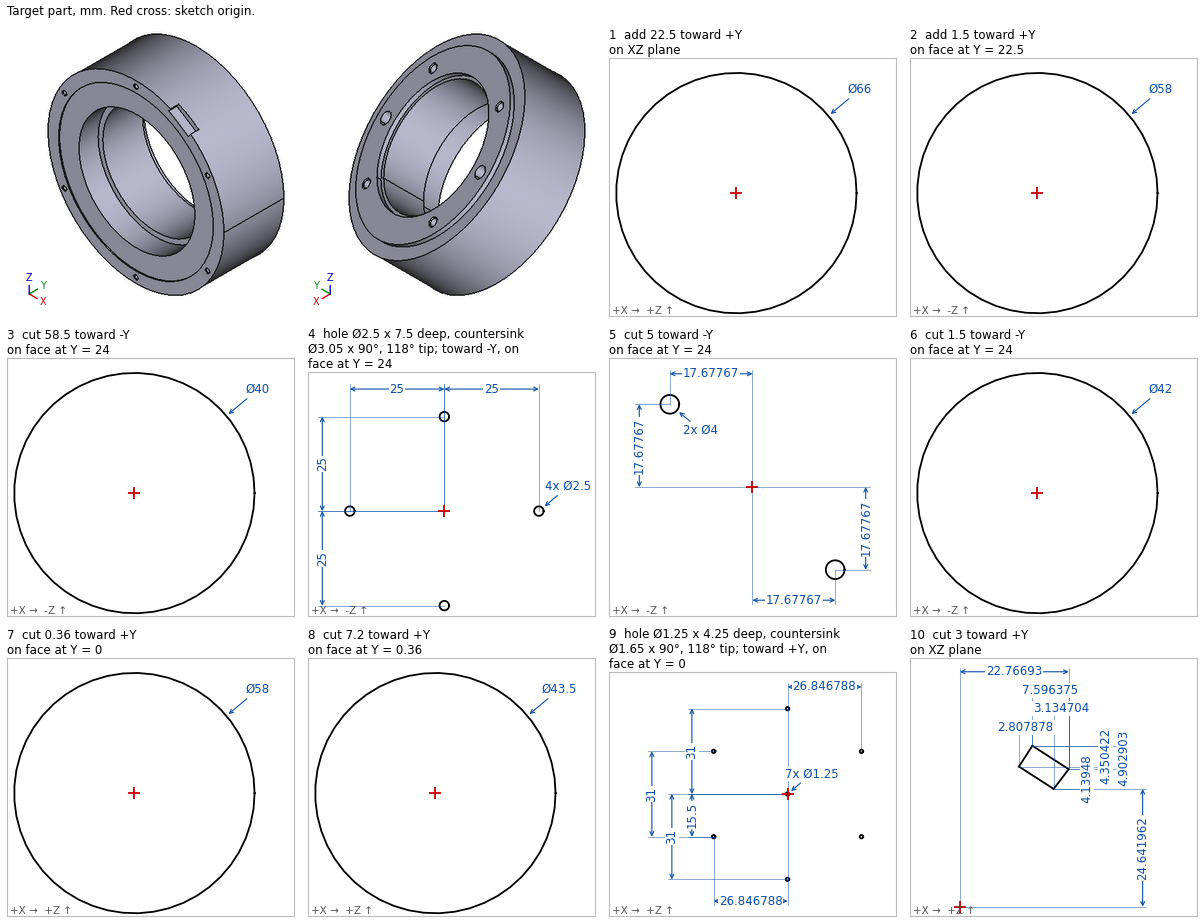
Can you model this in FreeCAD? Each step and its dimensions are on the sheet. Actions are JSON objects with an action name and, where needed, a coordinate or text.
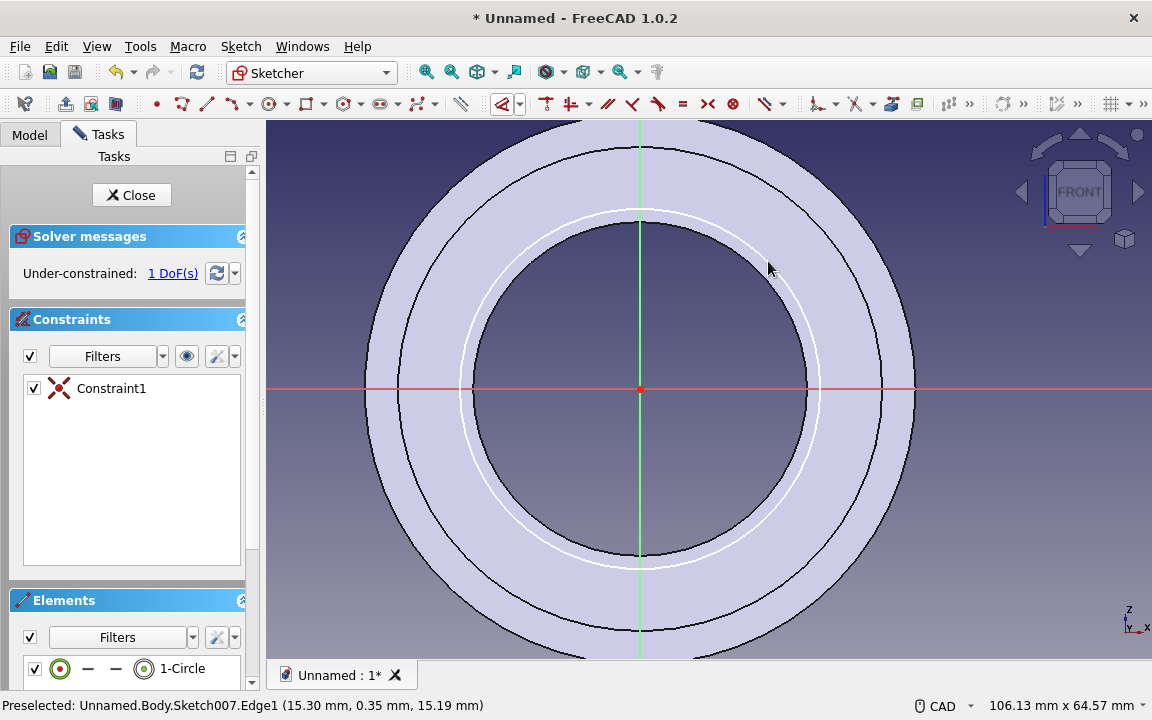
{"action": "left_click", "coordinate": [767, 261]}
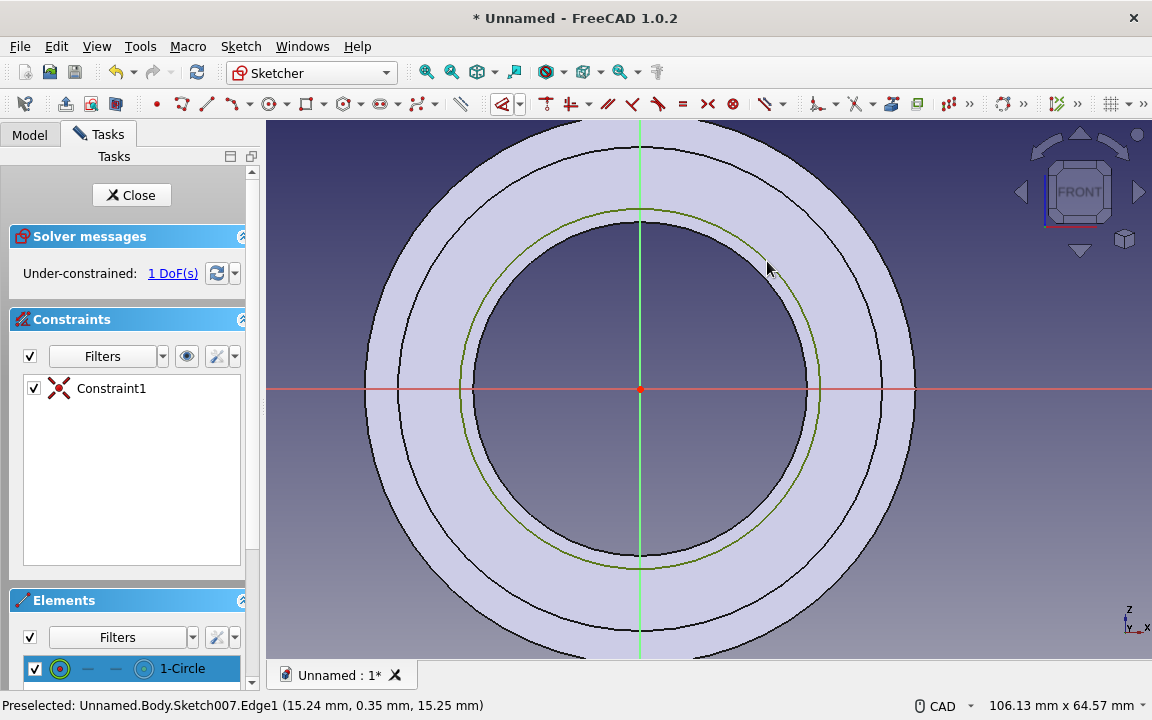
{"action": "left_click", "coordinate": [520, 104]}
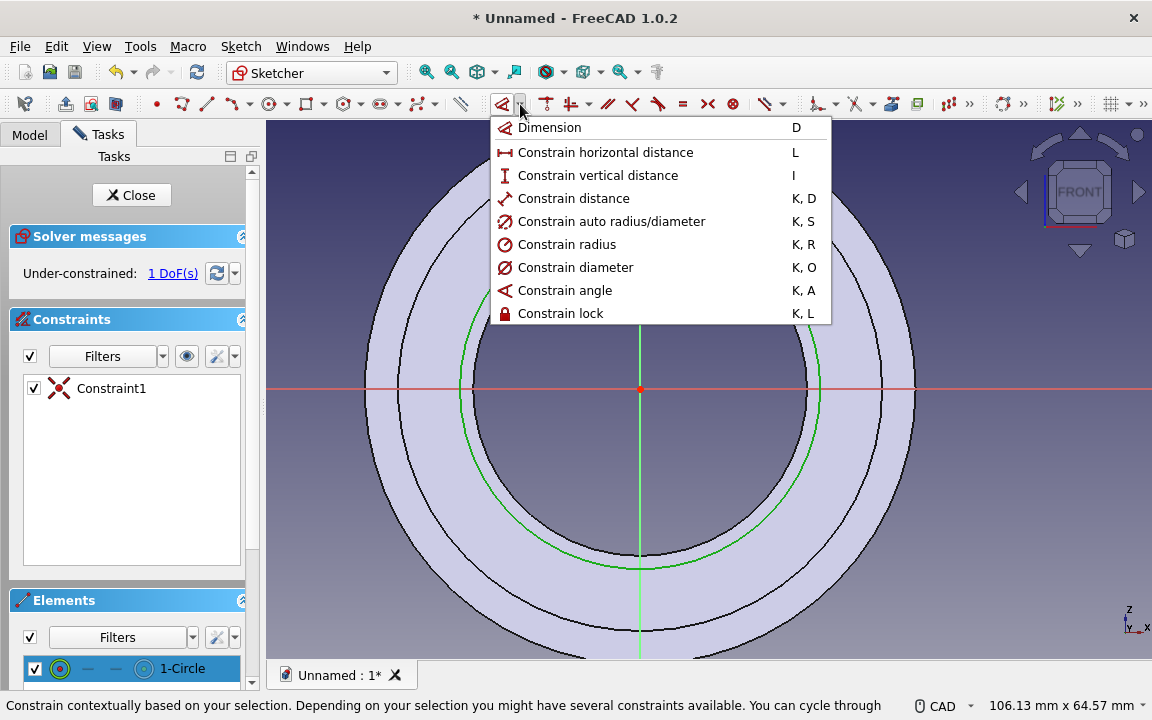
{"action": "left_click", "coordinate": [661, 268]}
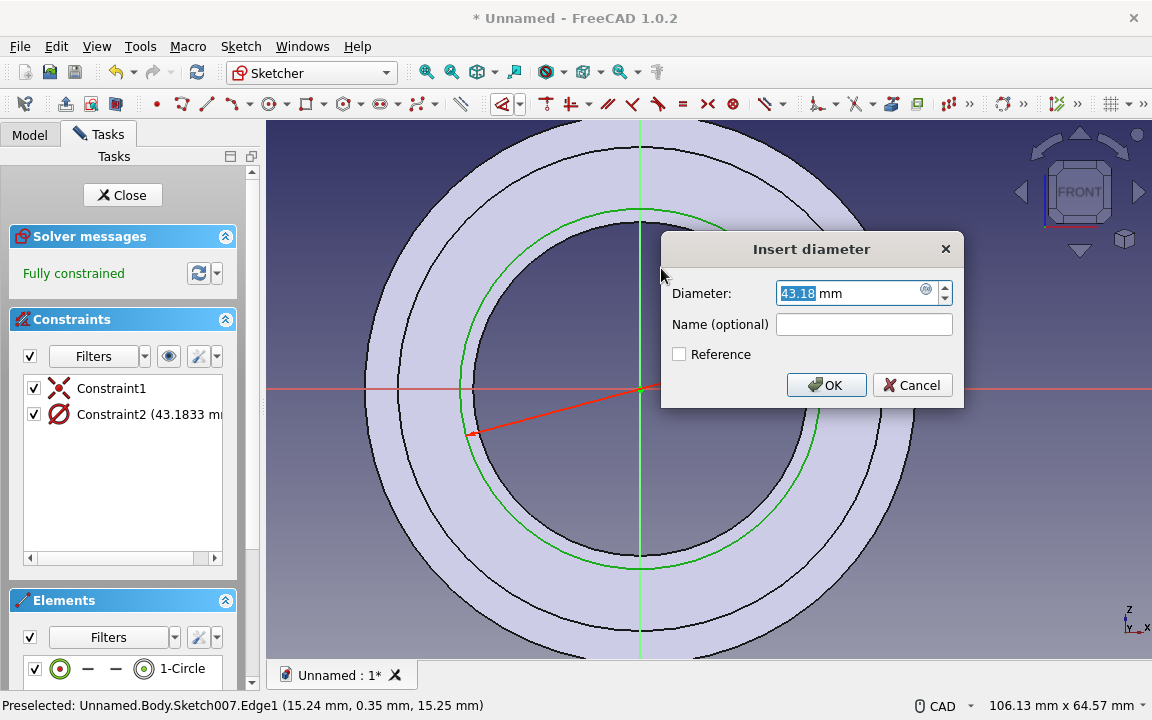
{"action": "type", "text": "43.5"}
{"action": "key", "text": "Return"}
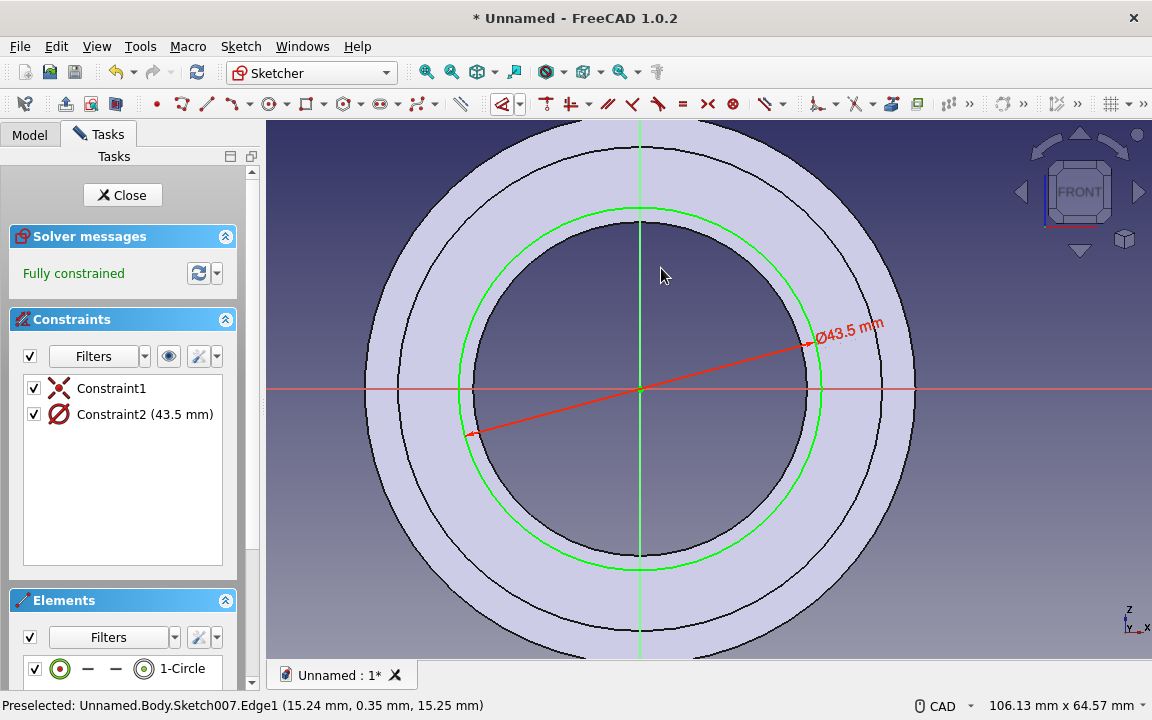
{"action": "left_click", "coordinate": [123, 195]}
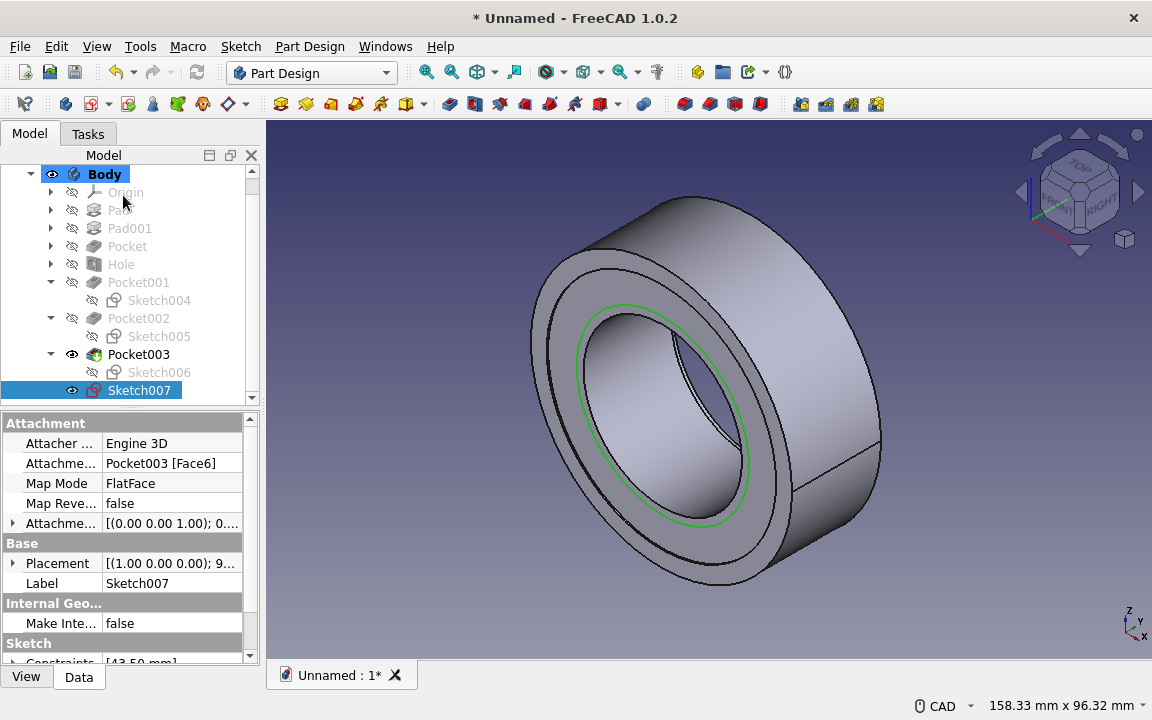
{"action": "left_click", "coordinate": [450, 104]}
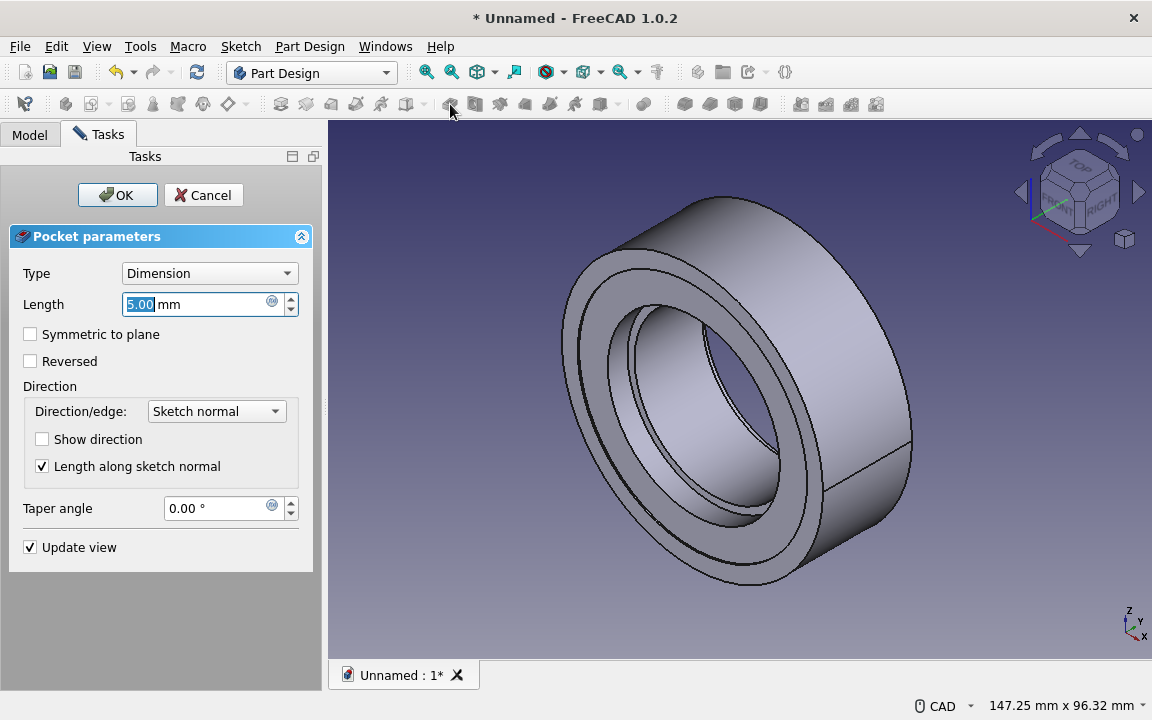
{"action": "type", "text": "7.2"}
{"action": "key", "text": "Tab"}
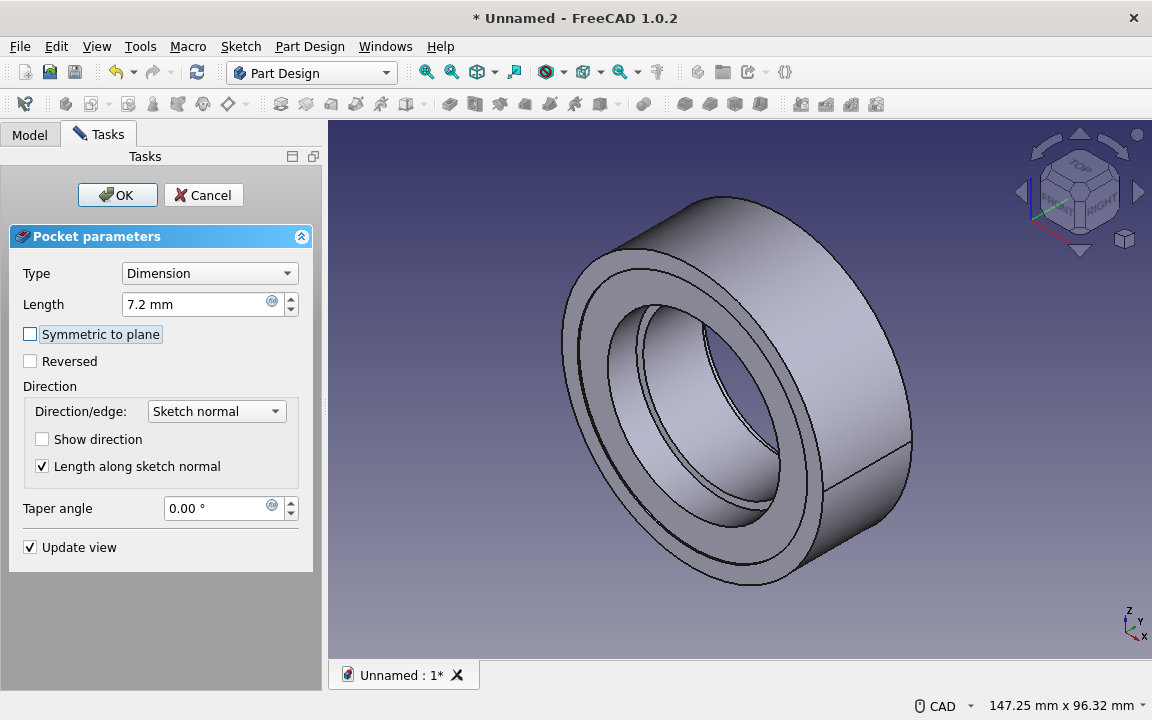
{"action": "left_click", "coordinate": [118, 195]}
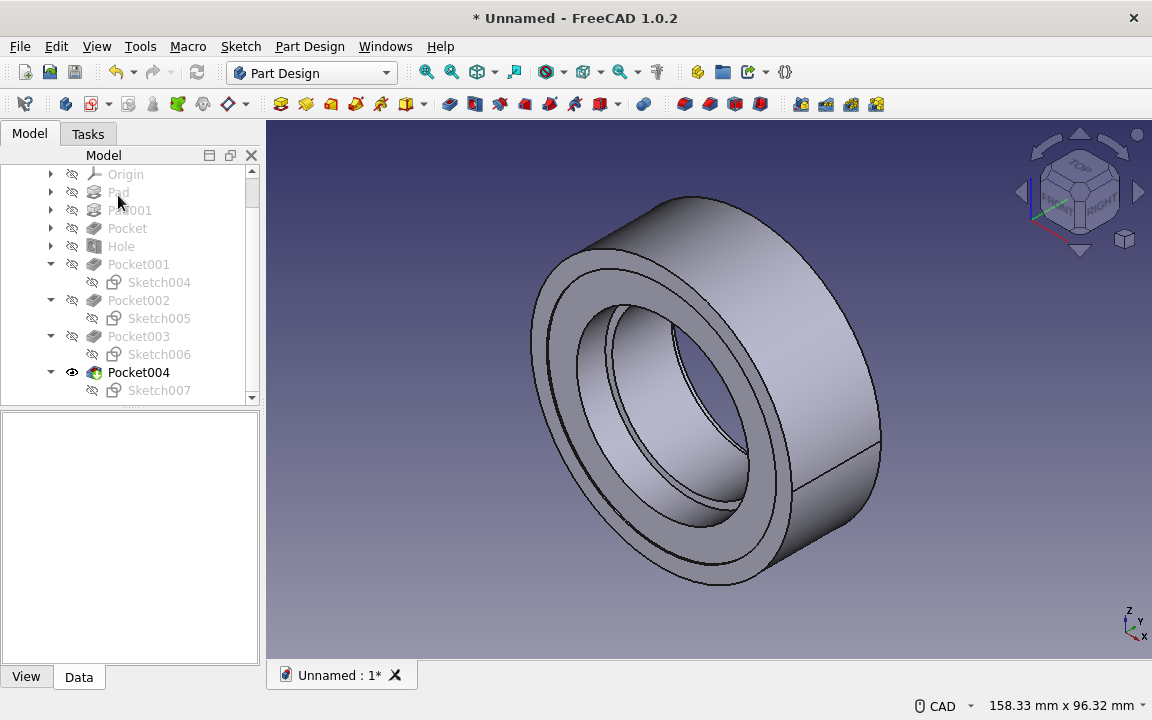
{"action": "left_click", "coordinate": [624, 265]}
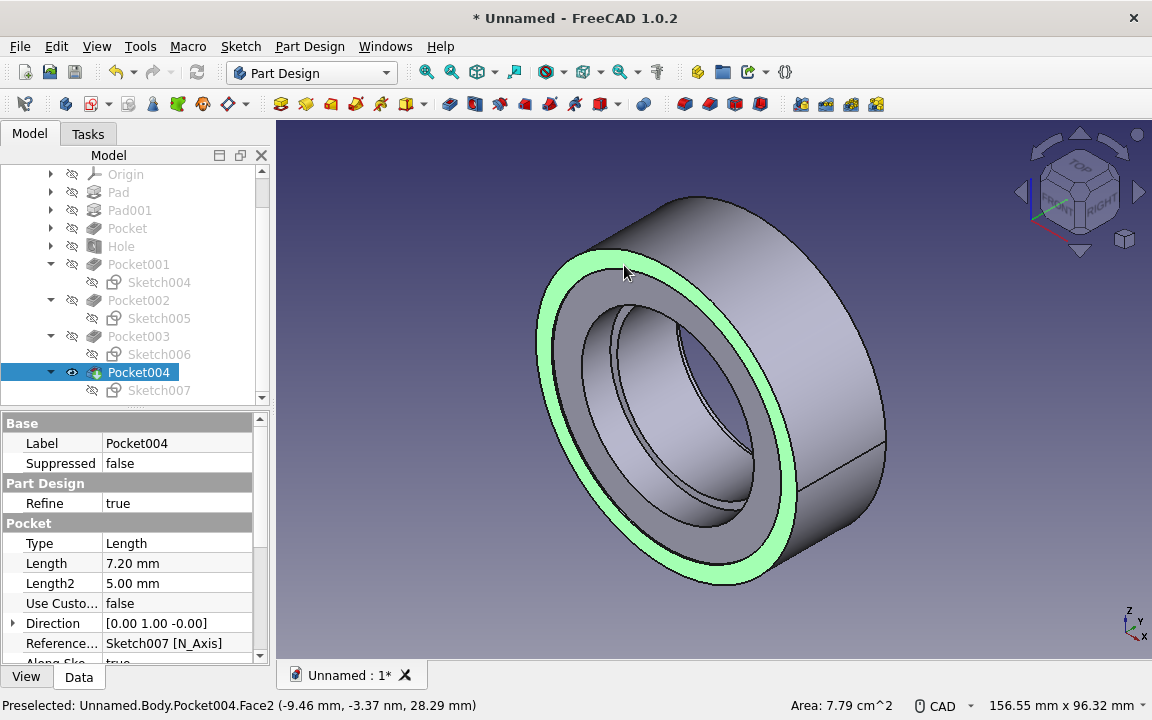
{"action": "left_click", "coordinate": [90, 104]}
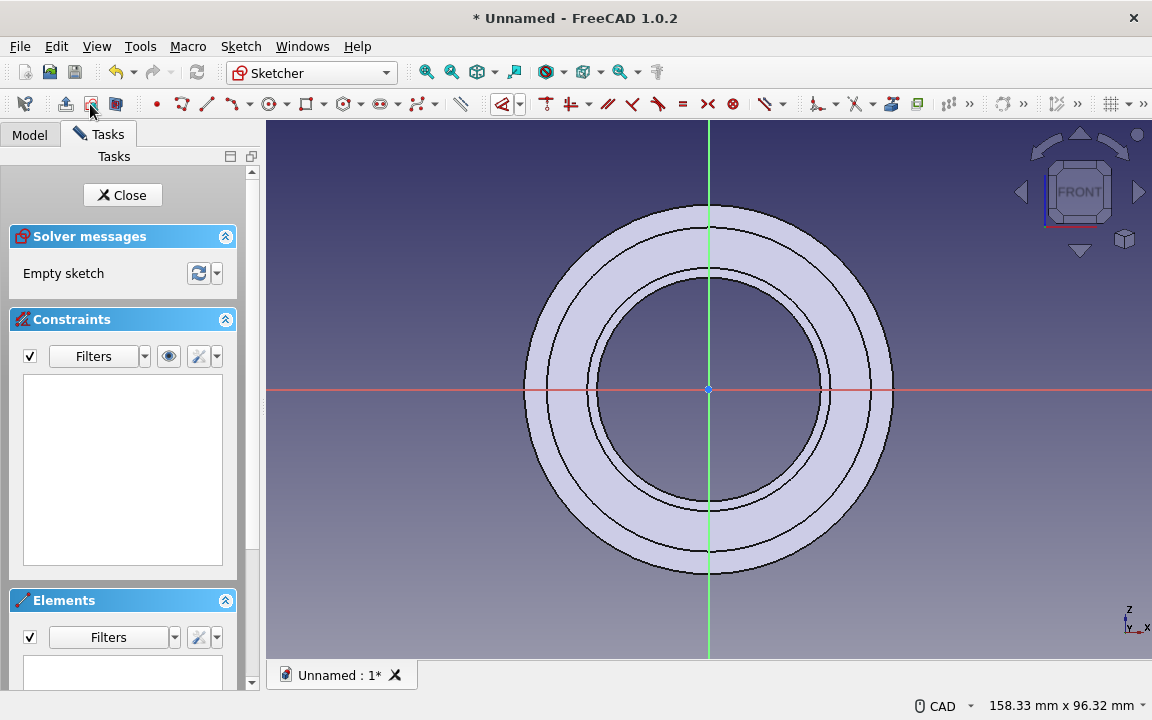
{"action": "left_click", "coordinate": [268, 104]}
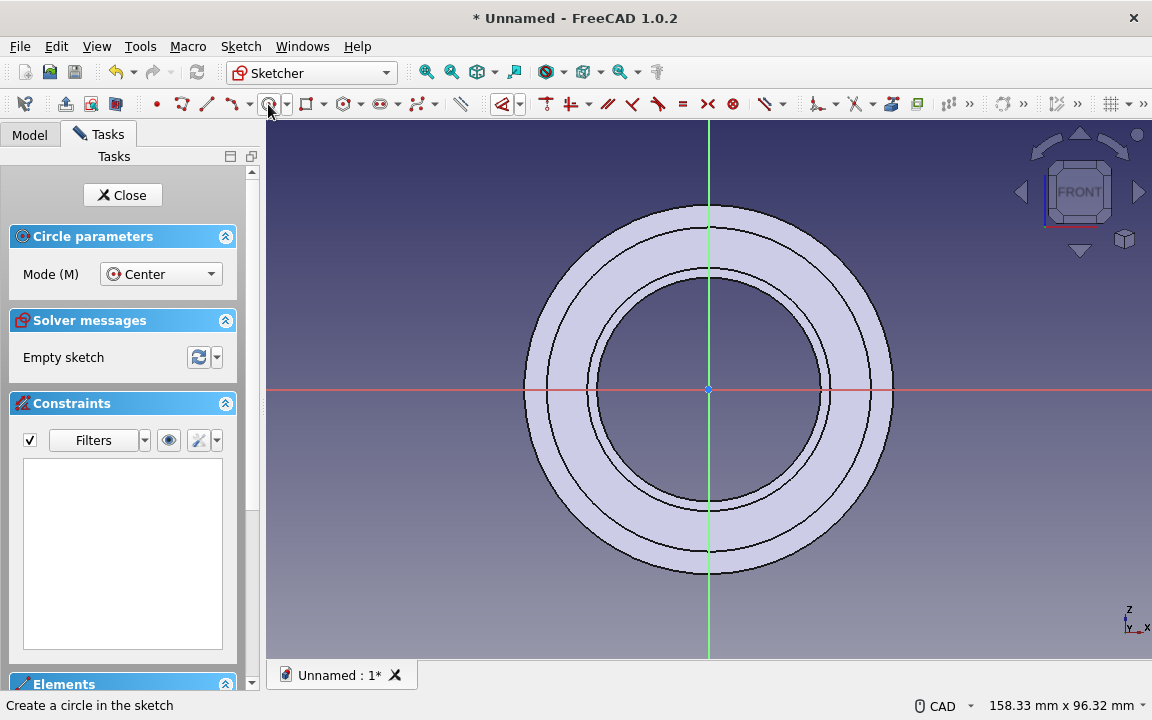
{"action": "scroll", "coordinate": [709, 390], "scroll_direction": "up", "scroll_amount": 10}